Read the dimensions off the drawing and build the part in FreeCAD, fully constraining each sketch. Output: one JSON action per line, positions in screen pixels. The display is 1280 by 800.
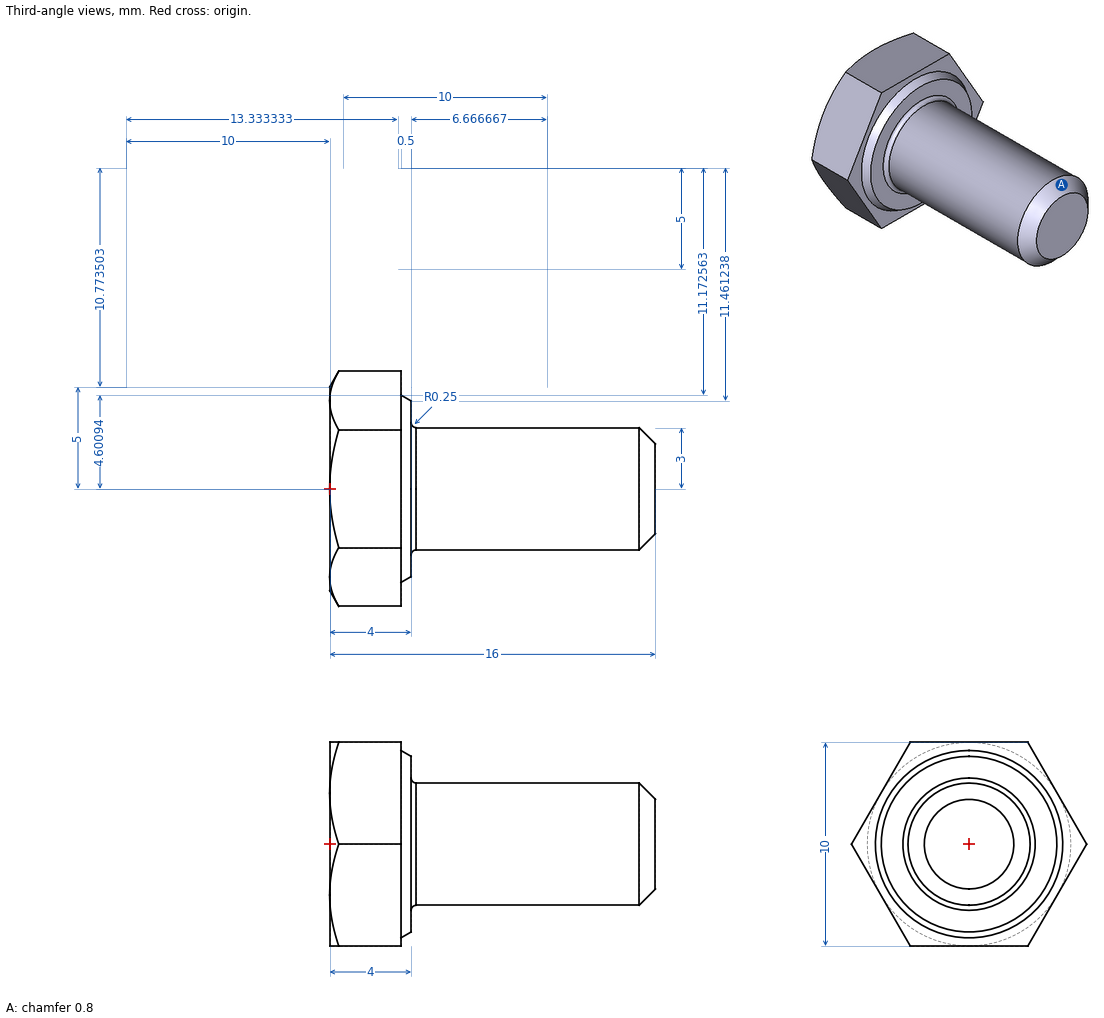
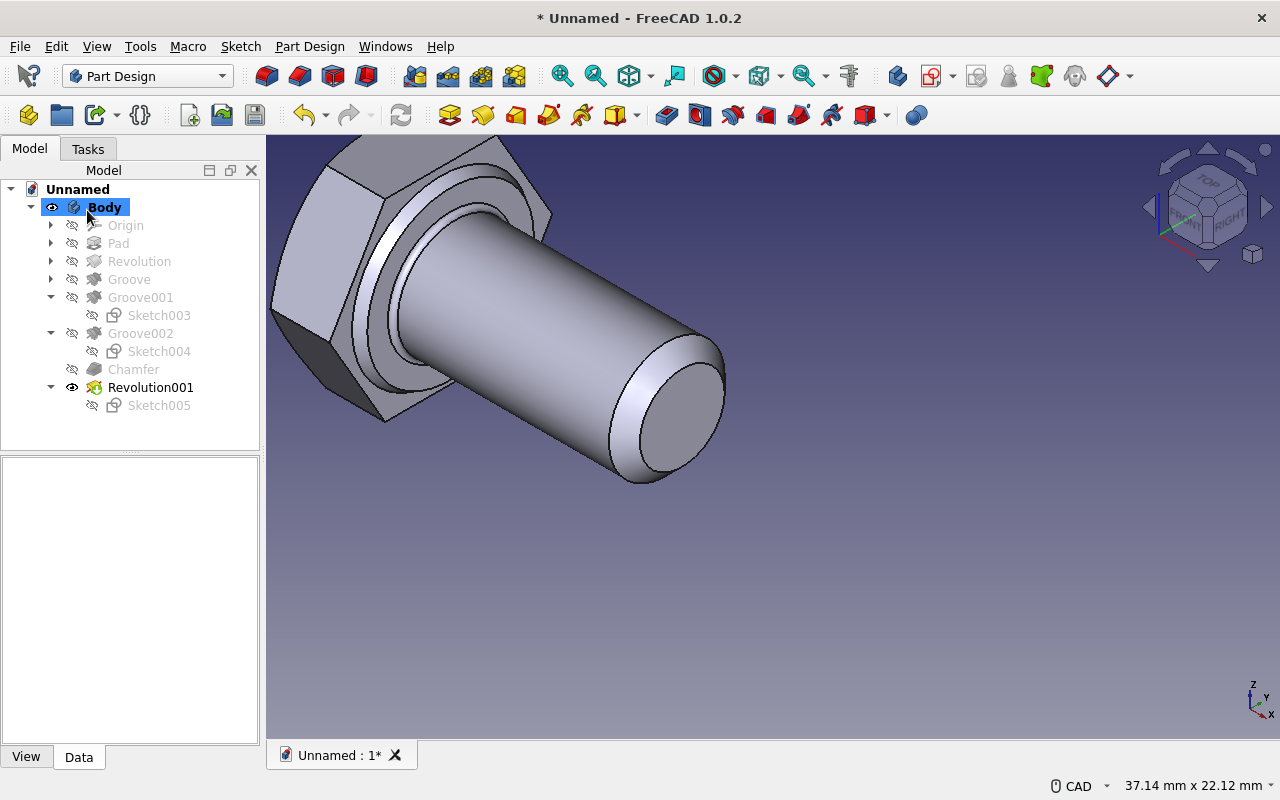
{"action": "left_click", "coordinate": [563, 76]}